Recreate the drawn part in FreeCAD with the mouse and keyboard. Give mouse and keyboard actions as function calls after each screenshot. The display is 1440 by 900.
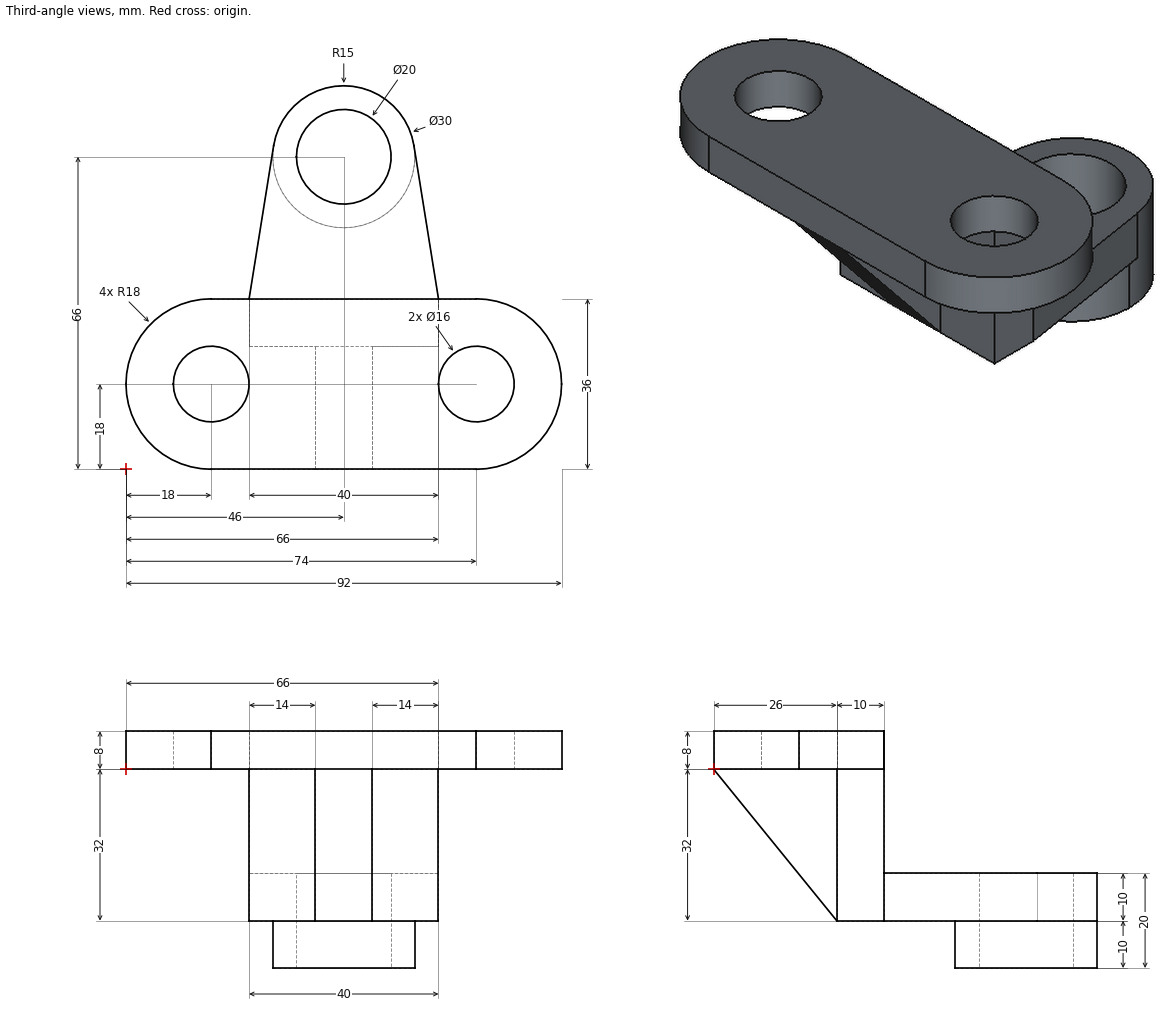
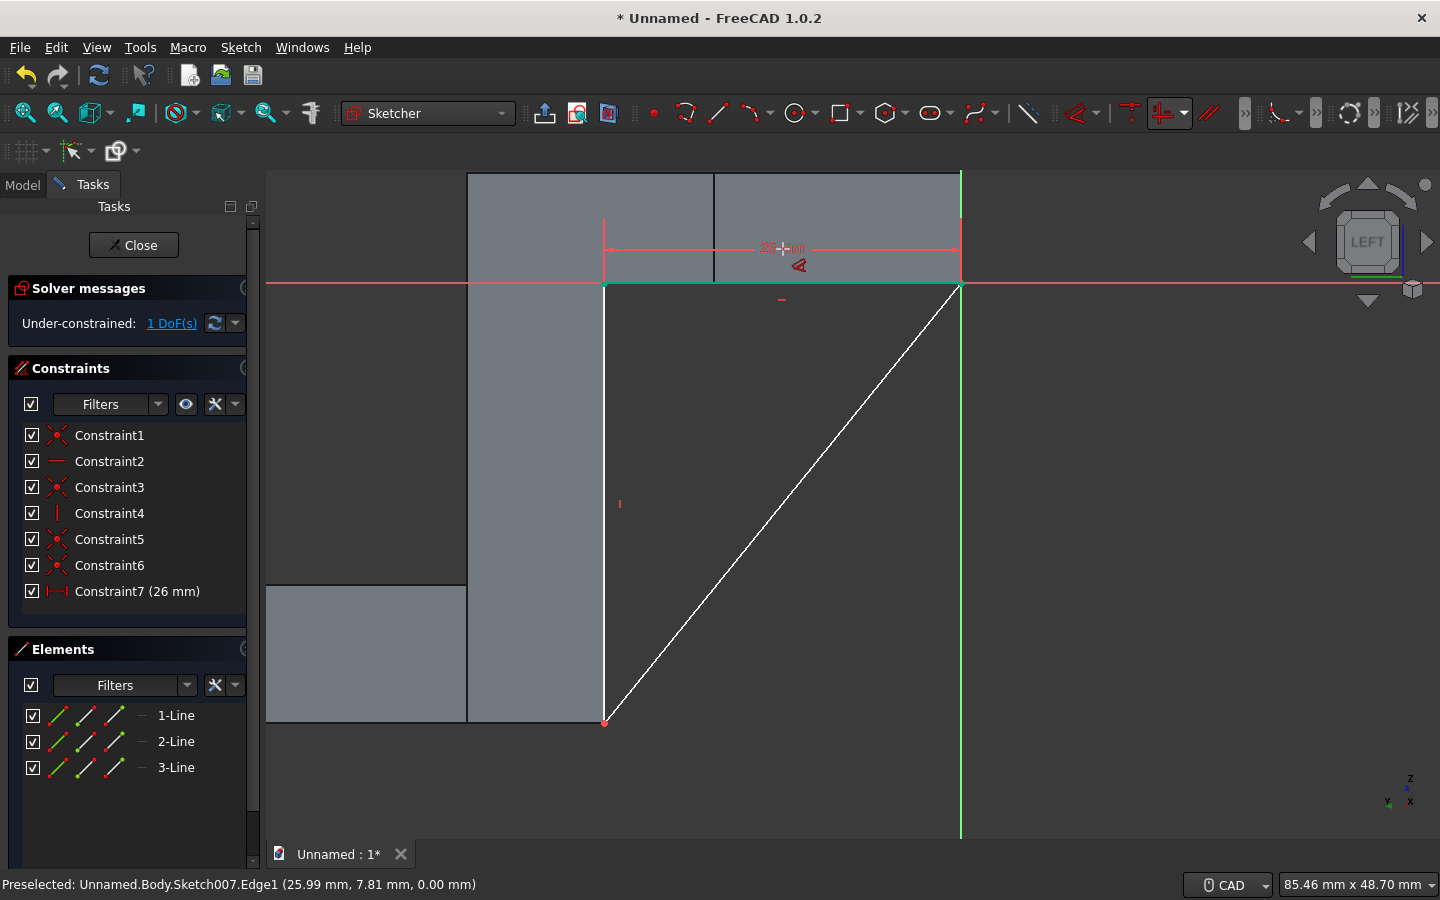
click(604, 415)
click(570, 504)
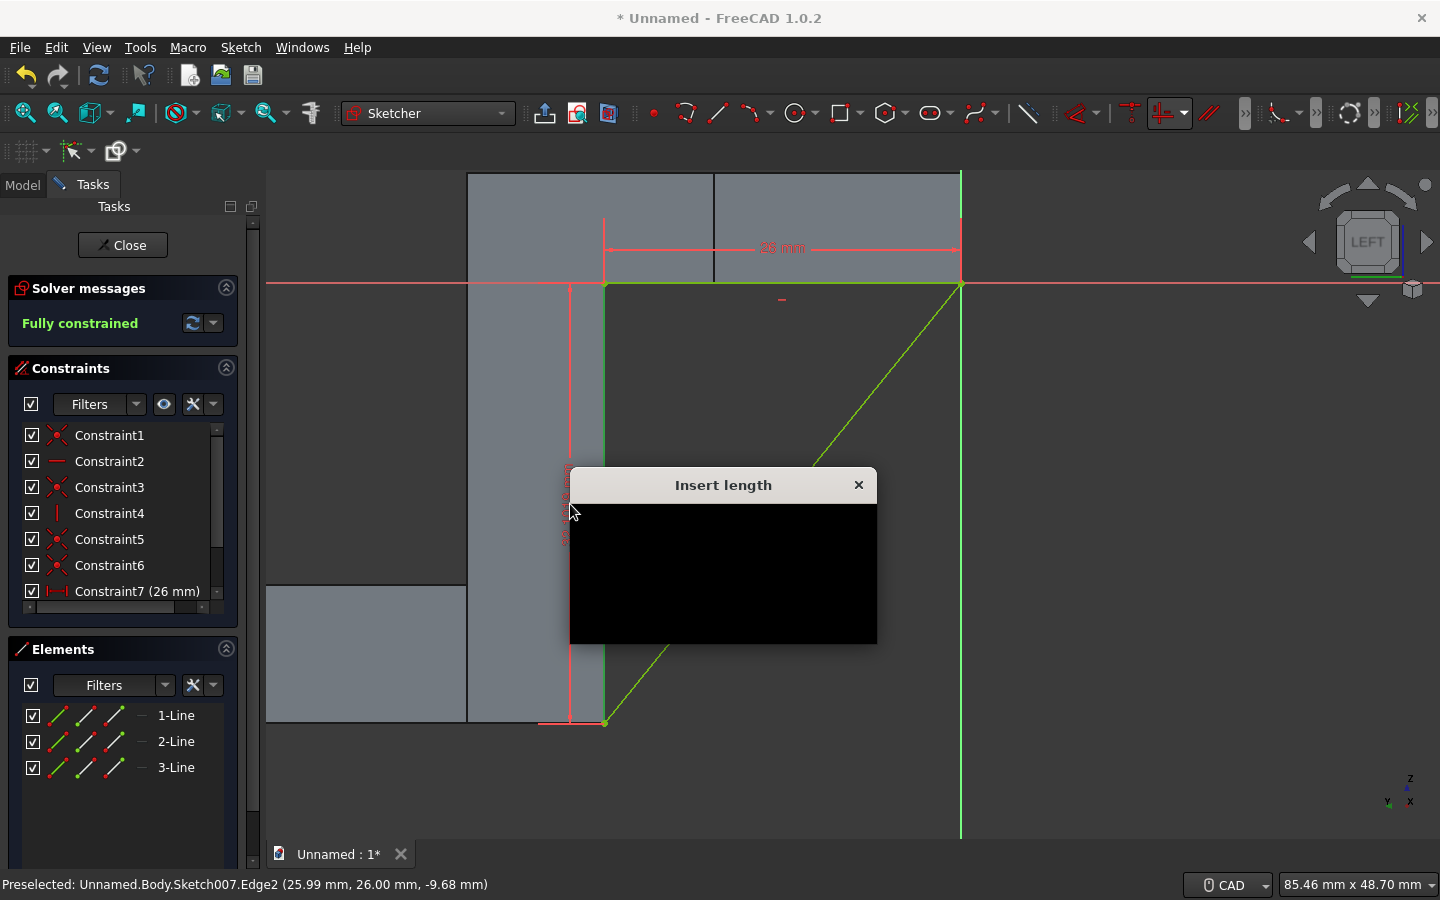
text(32)
key(Return)
key(Escape)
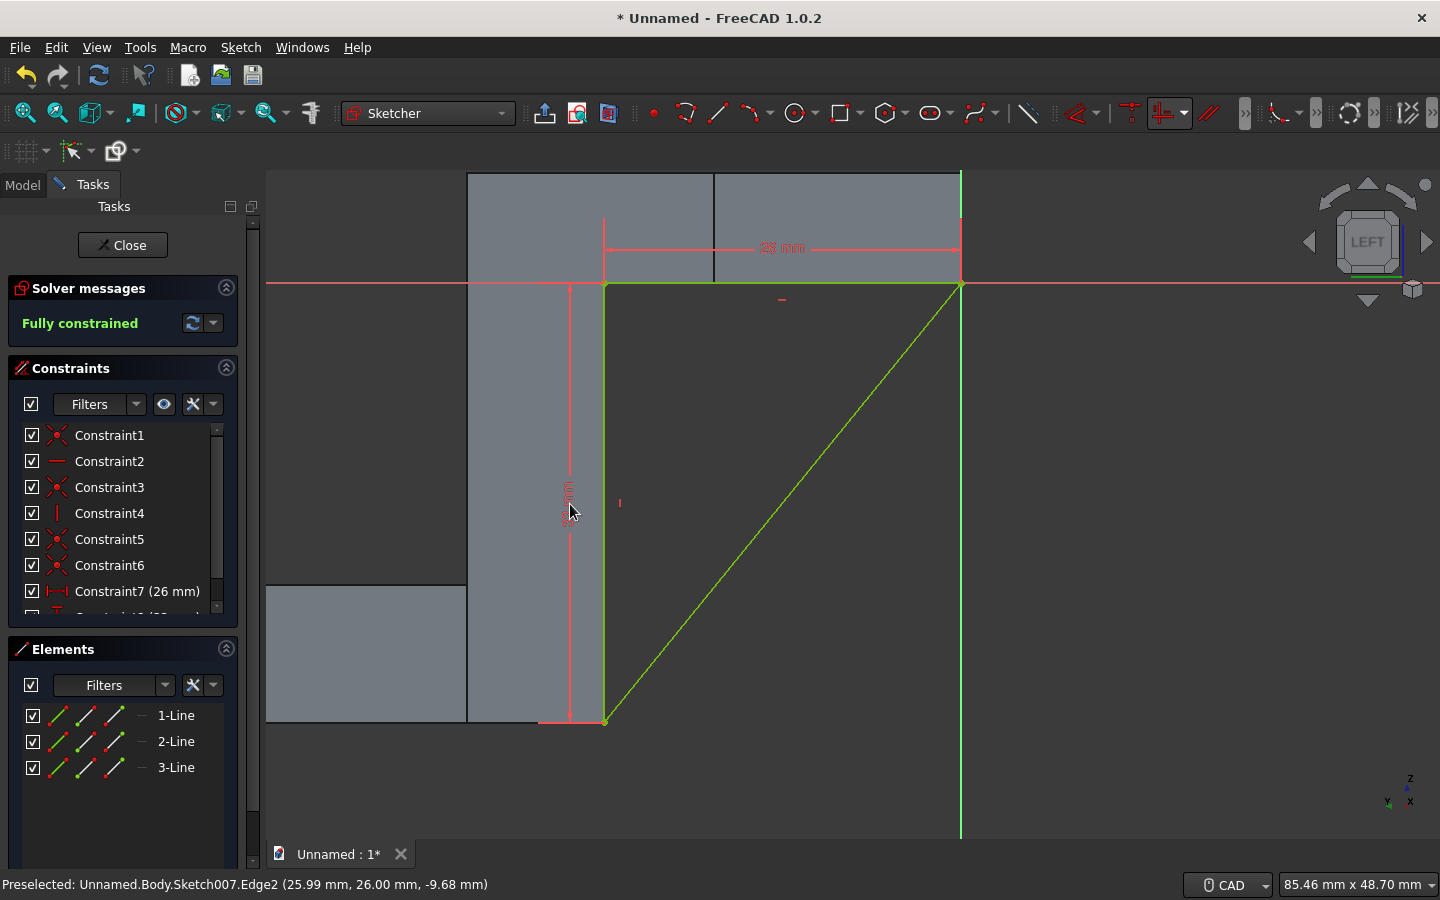
click(123, 245)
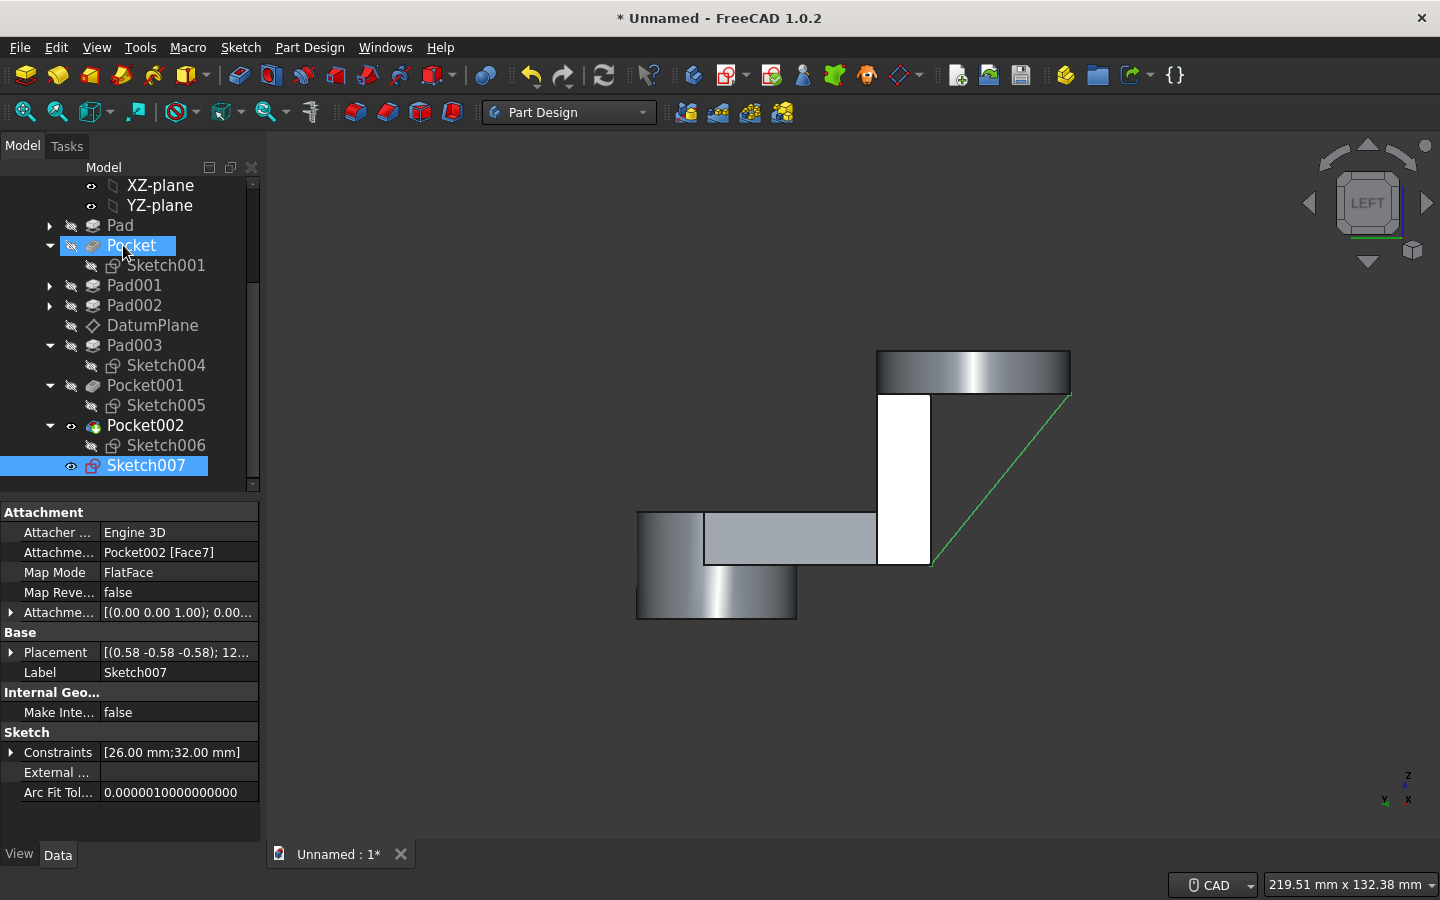
click(26, 76)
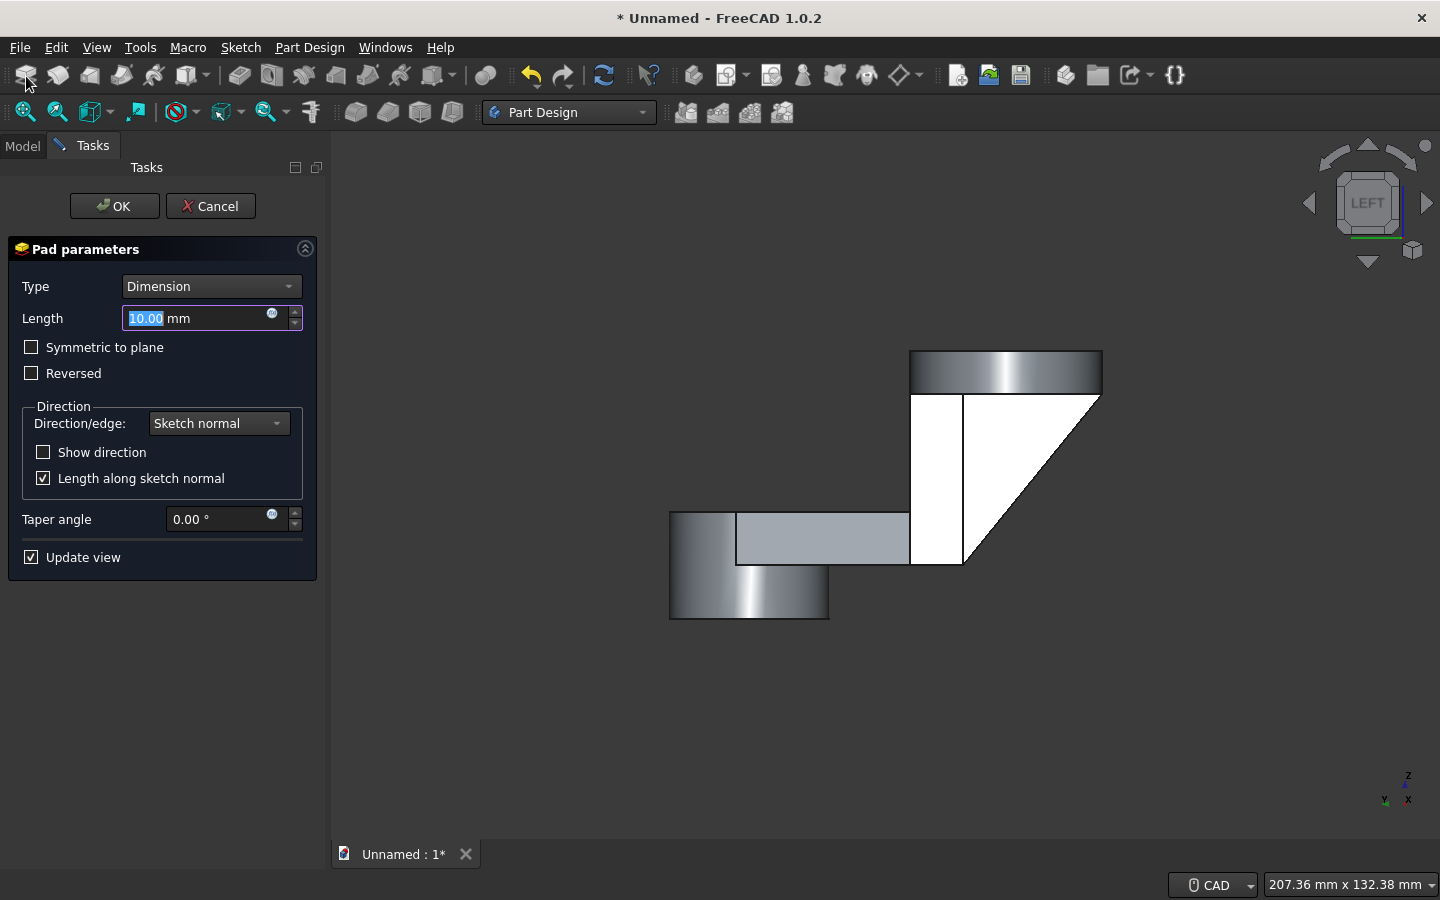
text(40)
key(Tab)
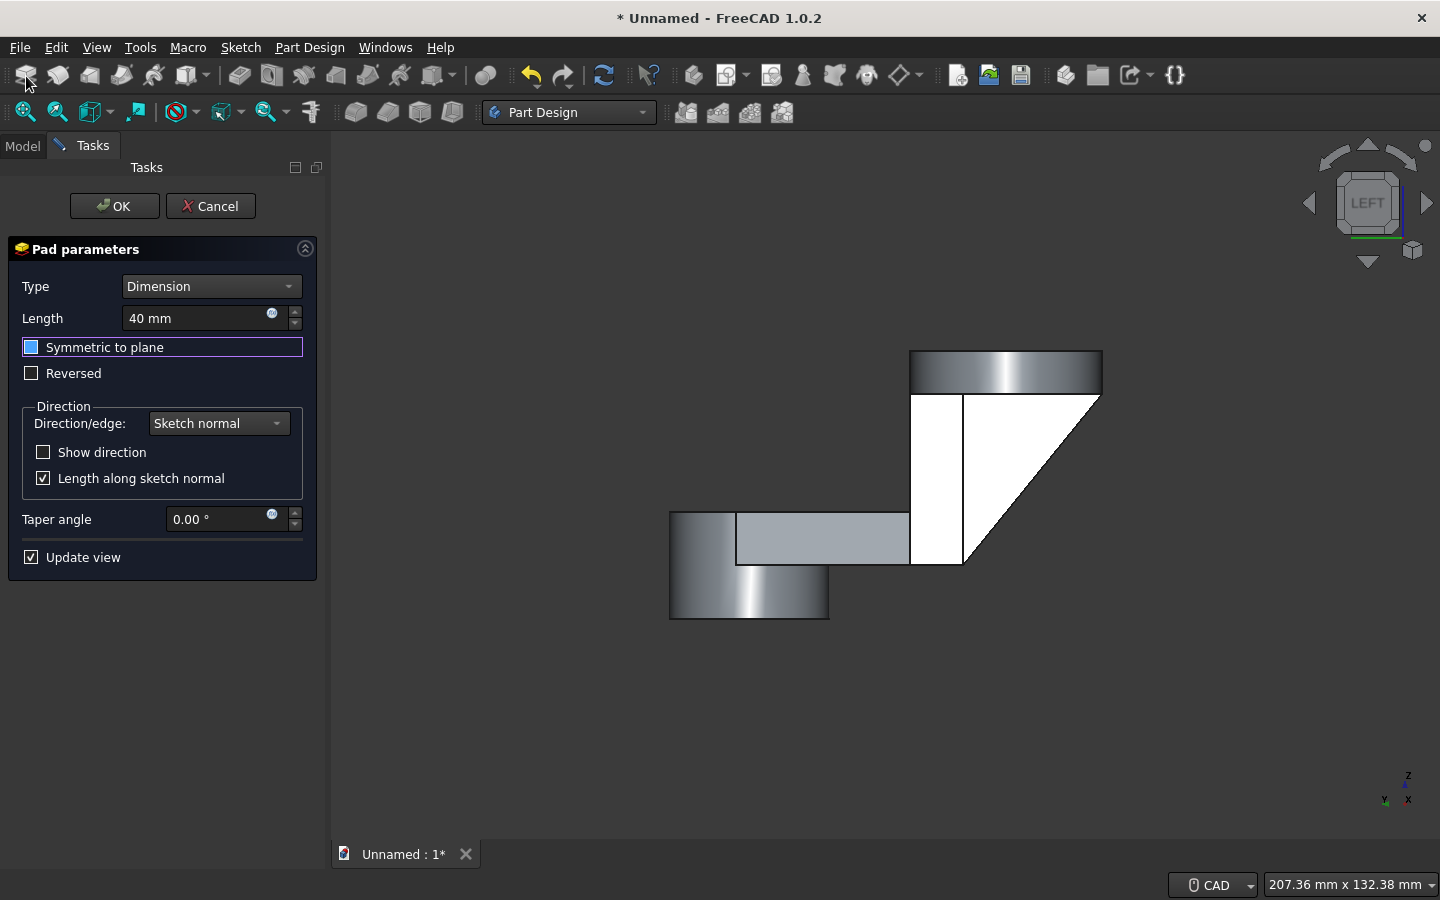
click(30, 373)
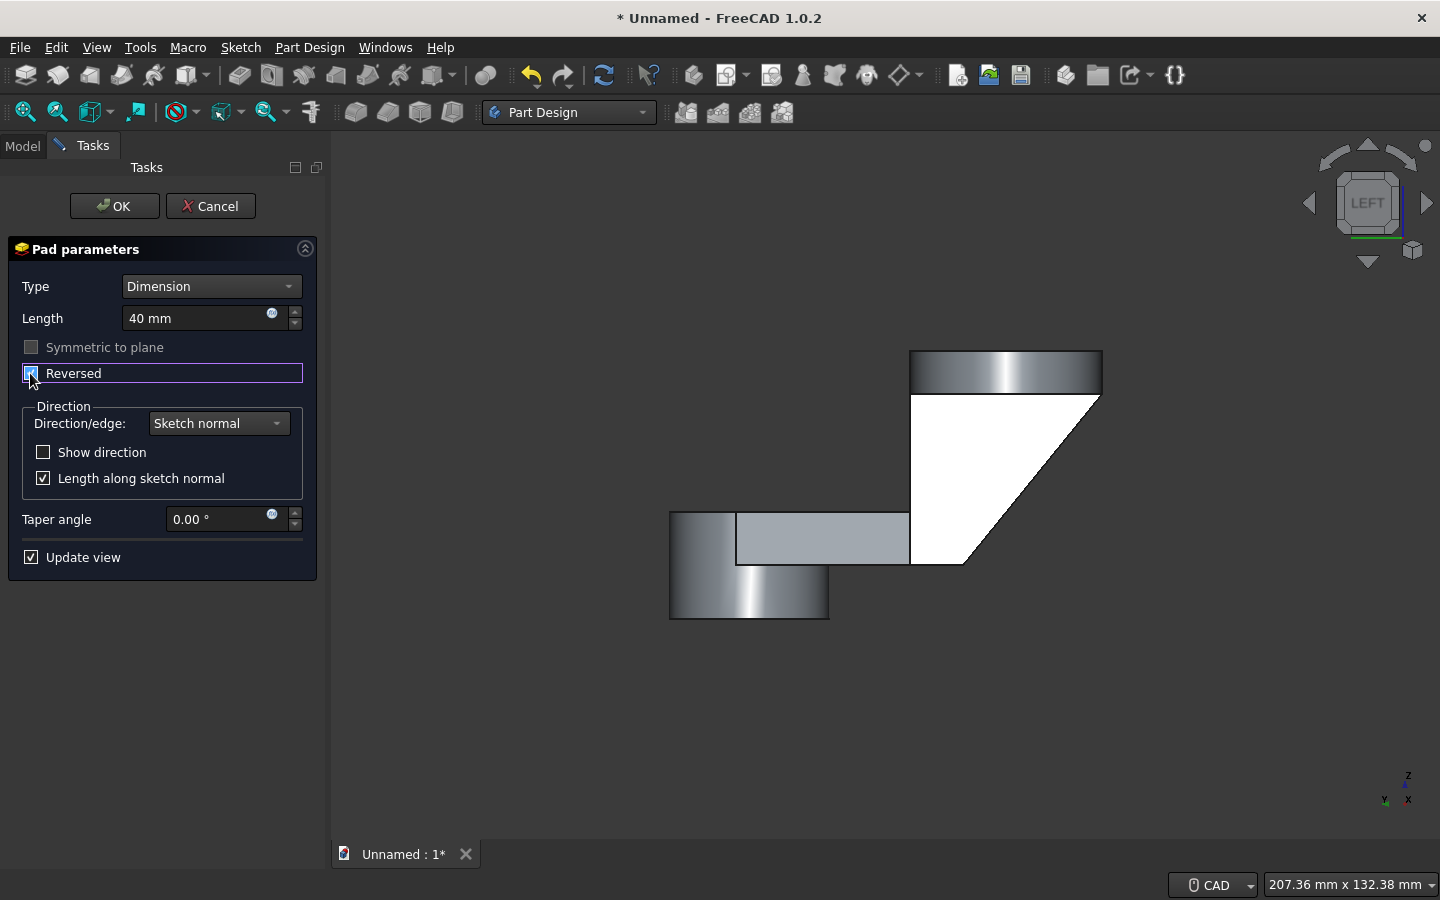
click(115, 206)